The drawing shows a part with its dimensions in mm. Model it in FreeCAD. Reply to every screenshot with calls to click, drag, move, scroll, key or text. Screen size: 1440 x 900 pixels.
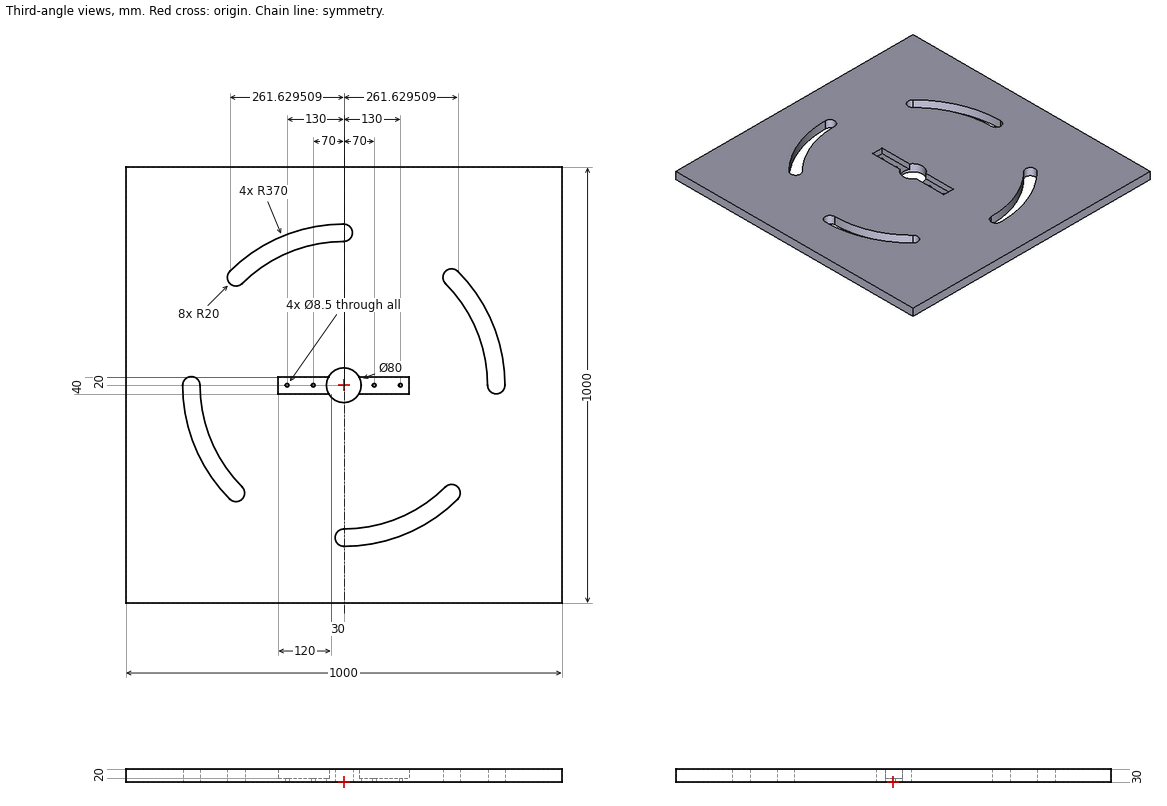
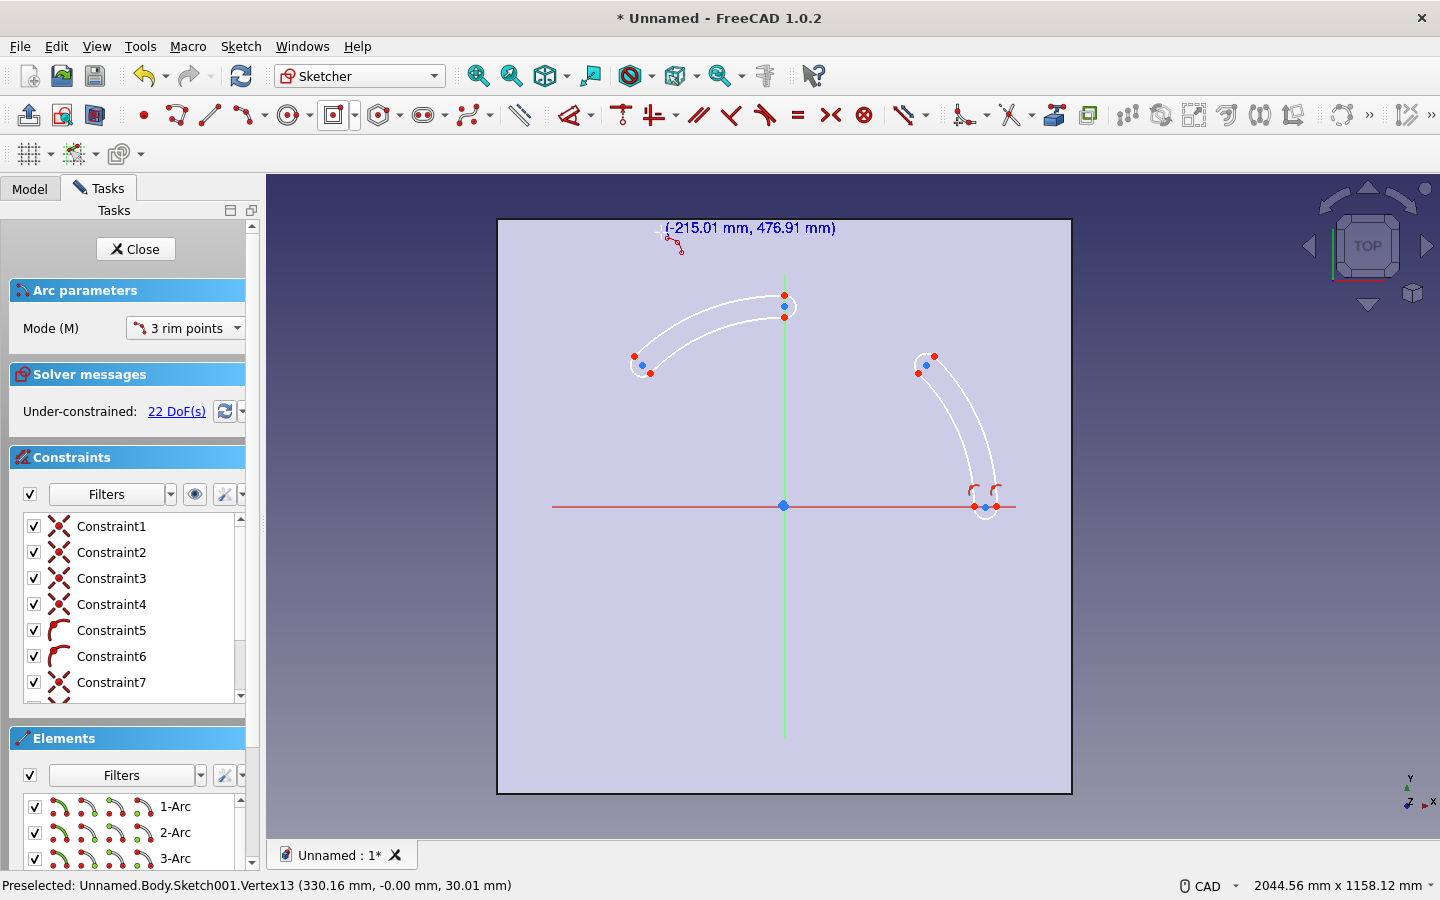
click(785, 696)
click(785, 719)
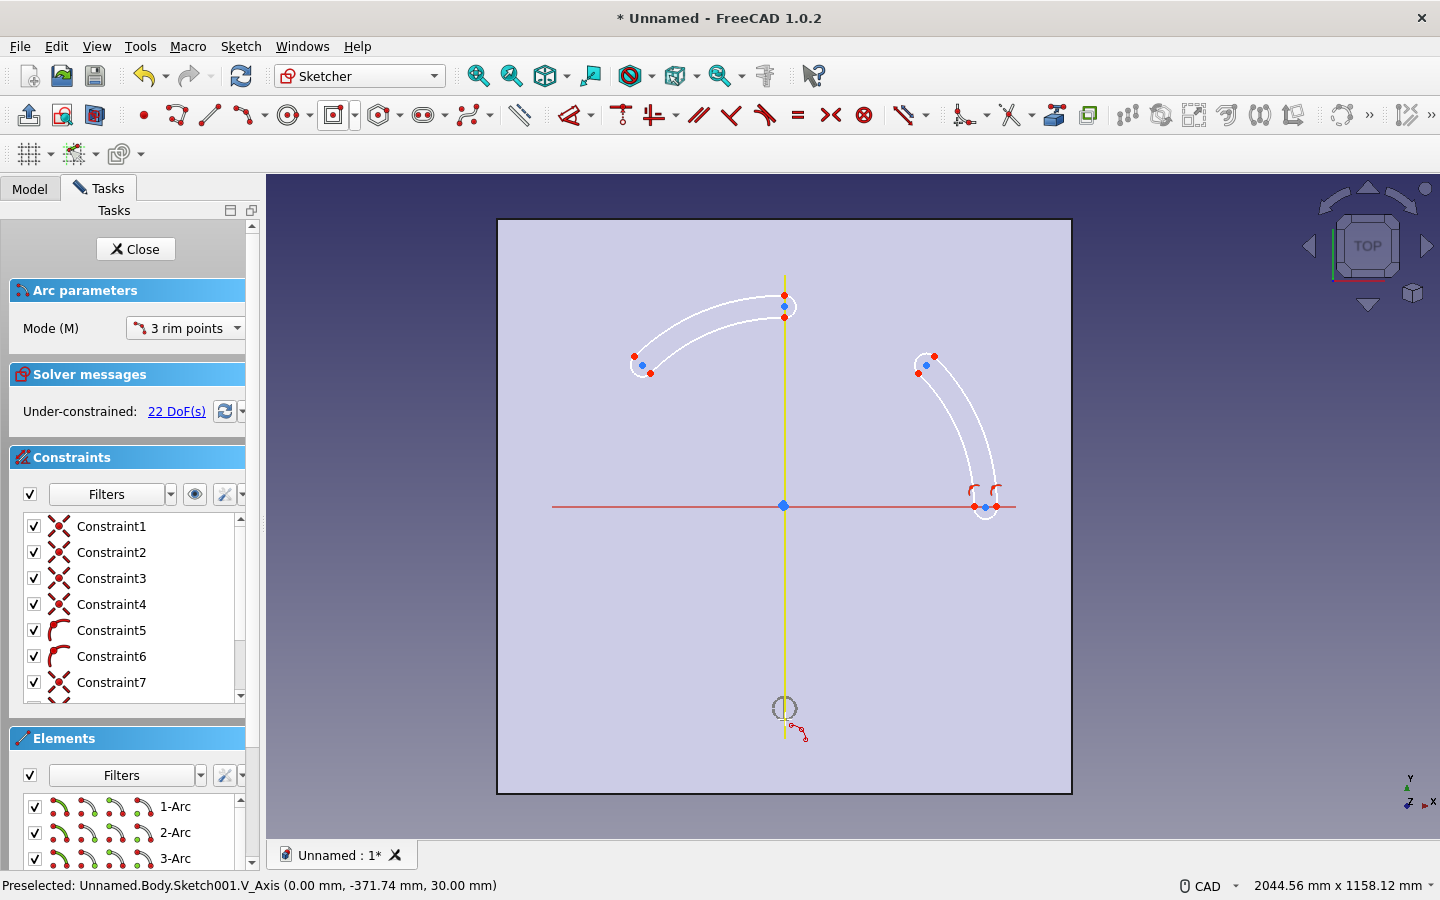
scroll(773, 708, up, 2)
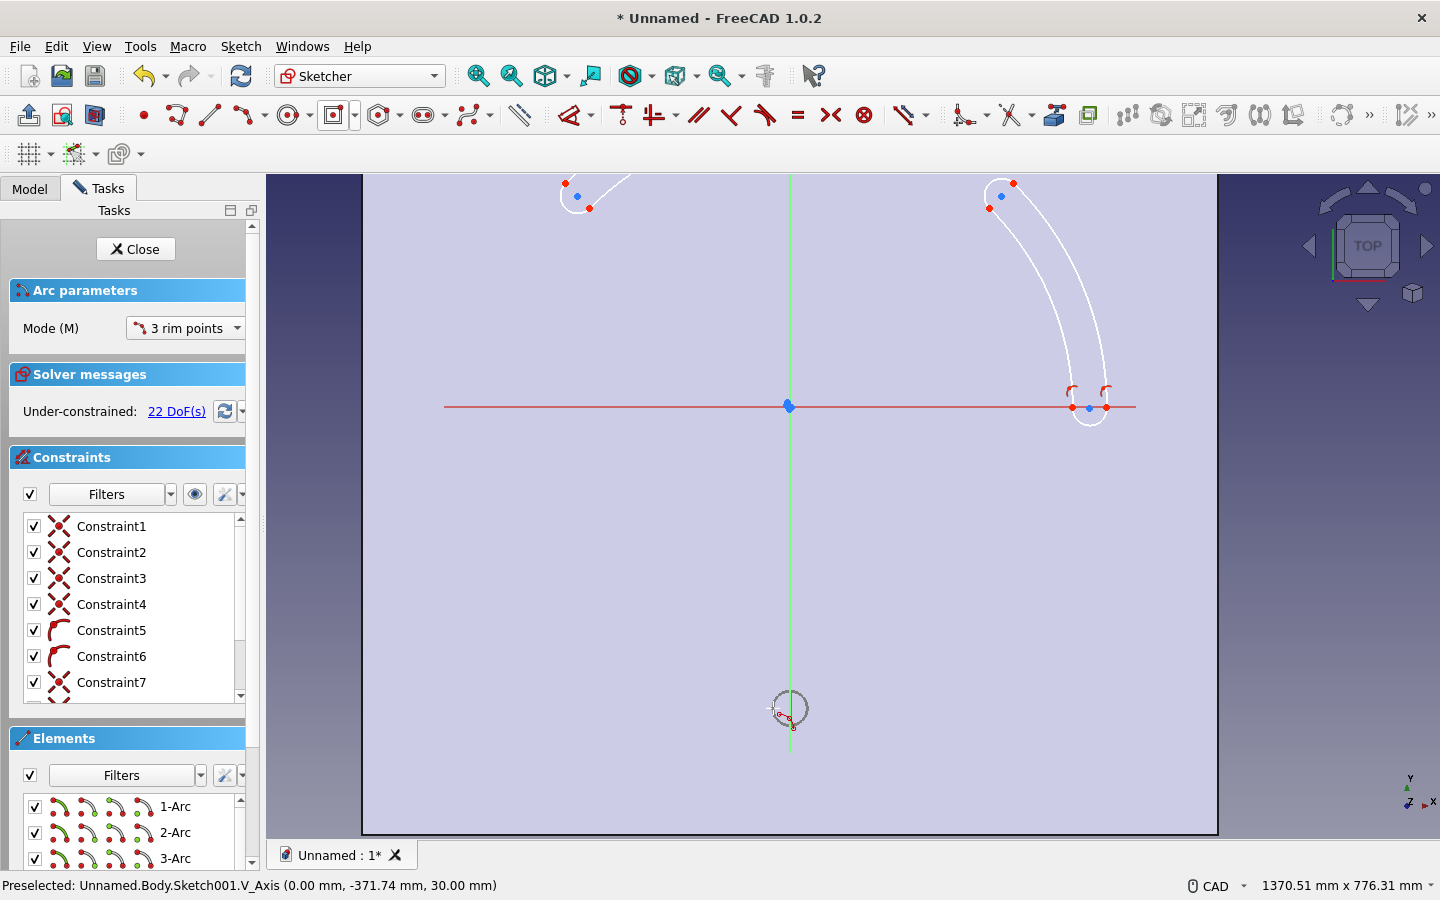
click(773, 707)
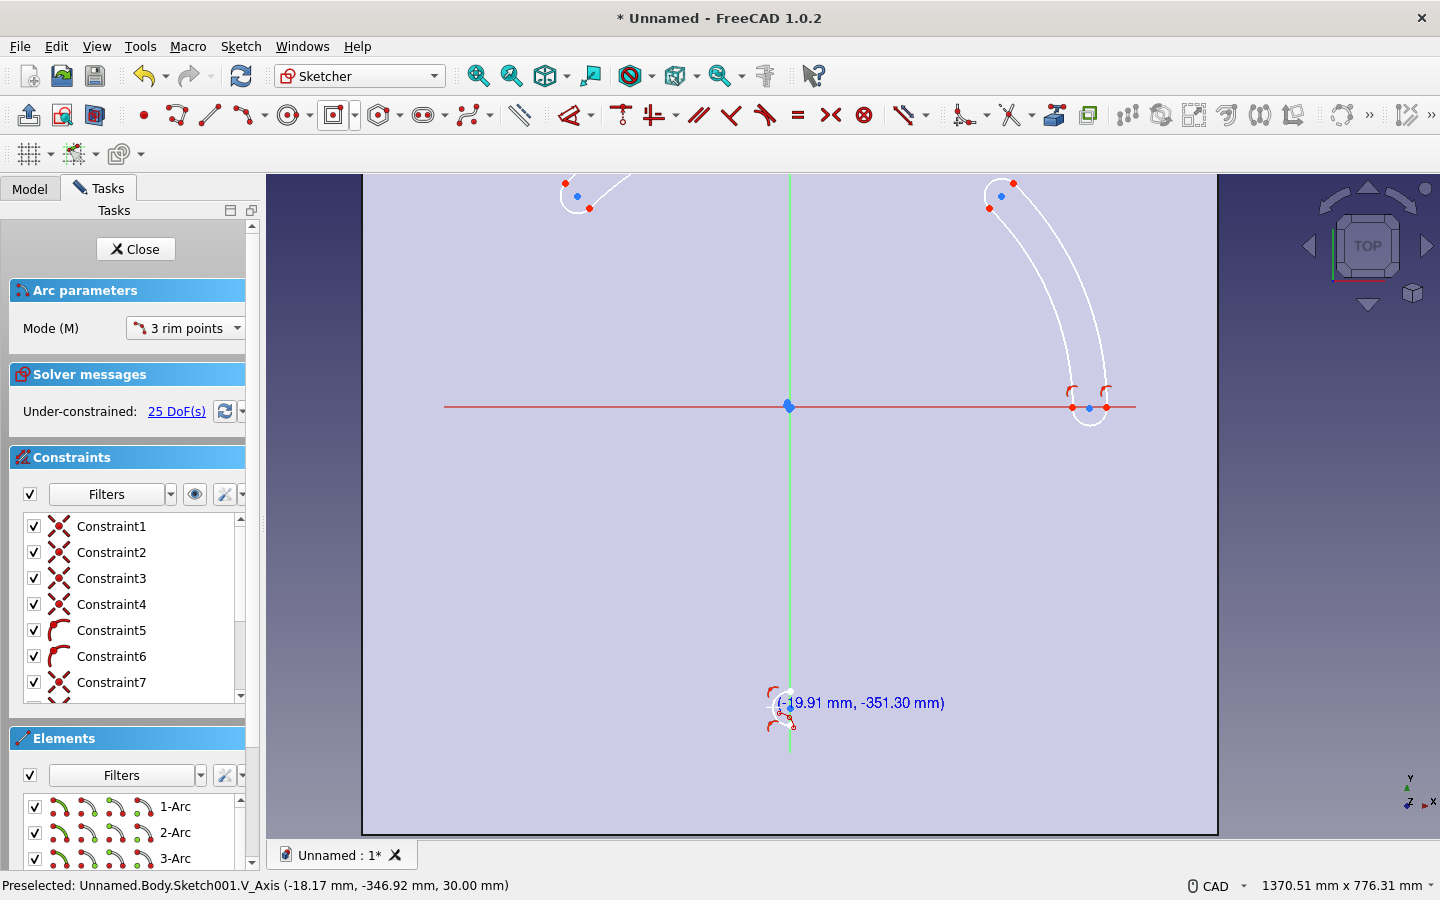
click(790, 726)
click(1014, 631)
click(911, 700)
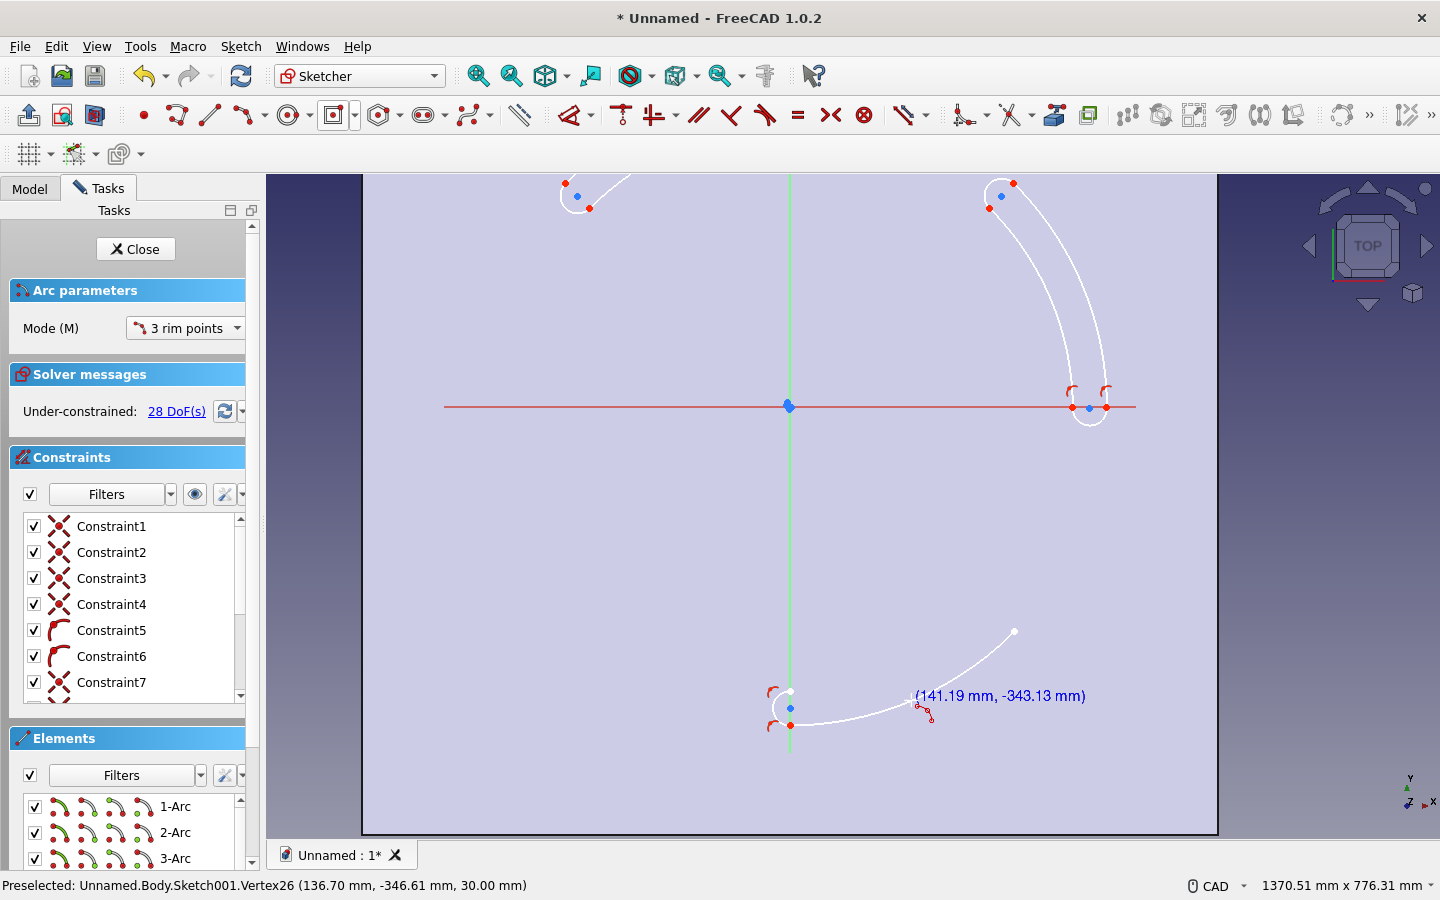
click(1014, 632)
click(990, 607)
click(1014, 607)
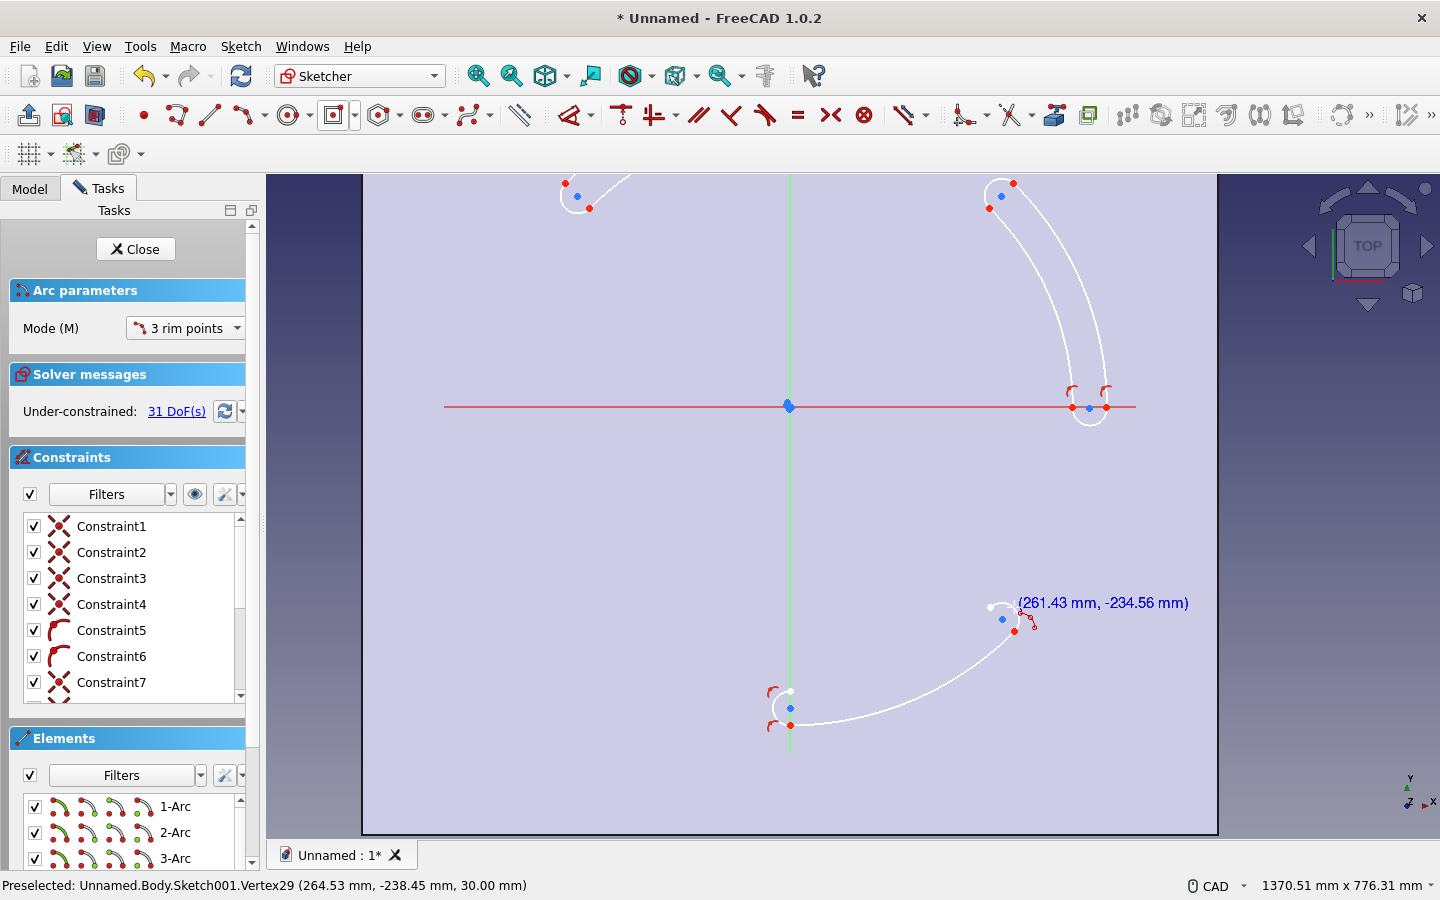
click(990, 608)
click(790, 691)
click(898, 668)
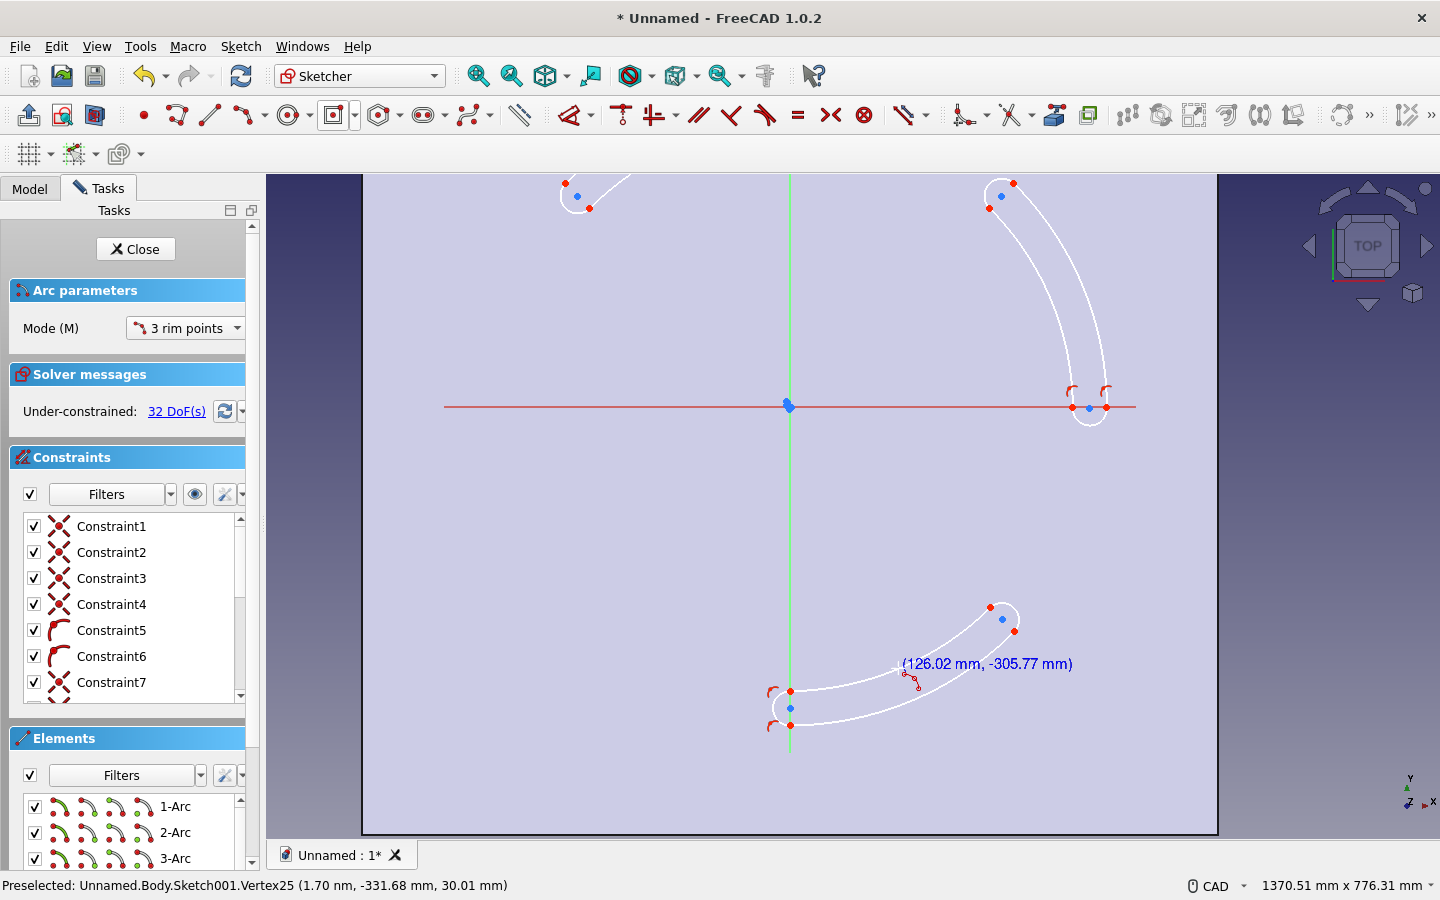
click(507, 407)
click(473, 407)
click(490, 390)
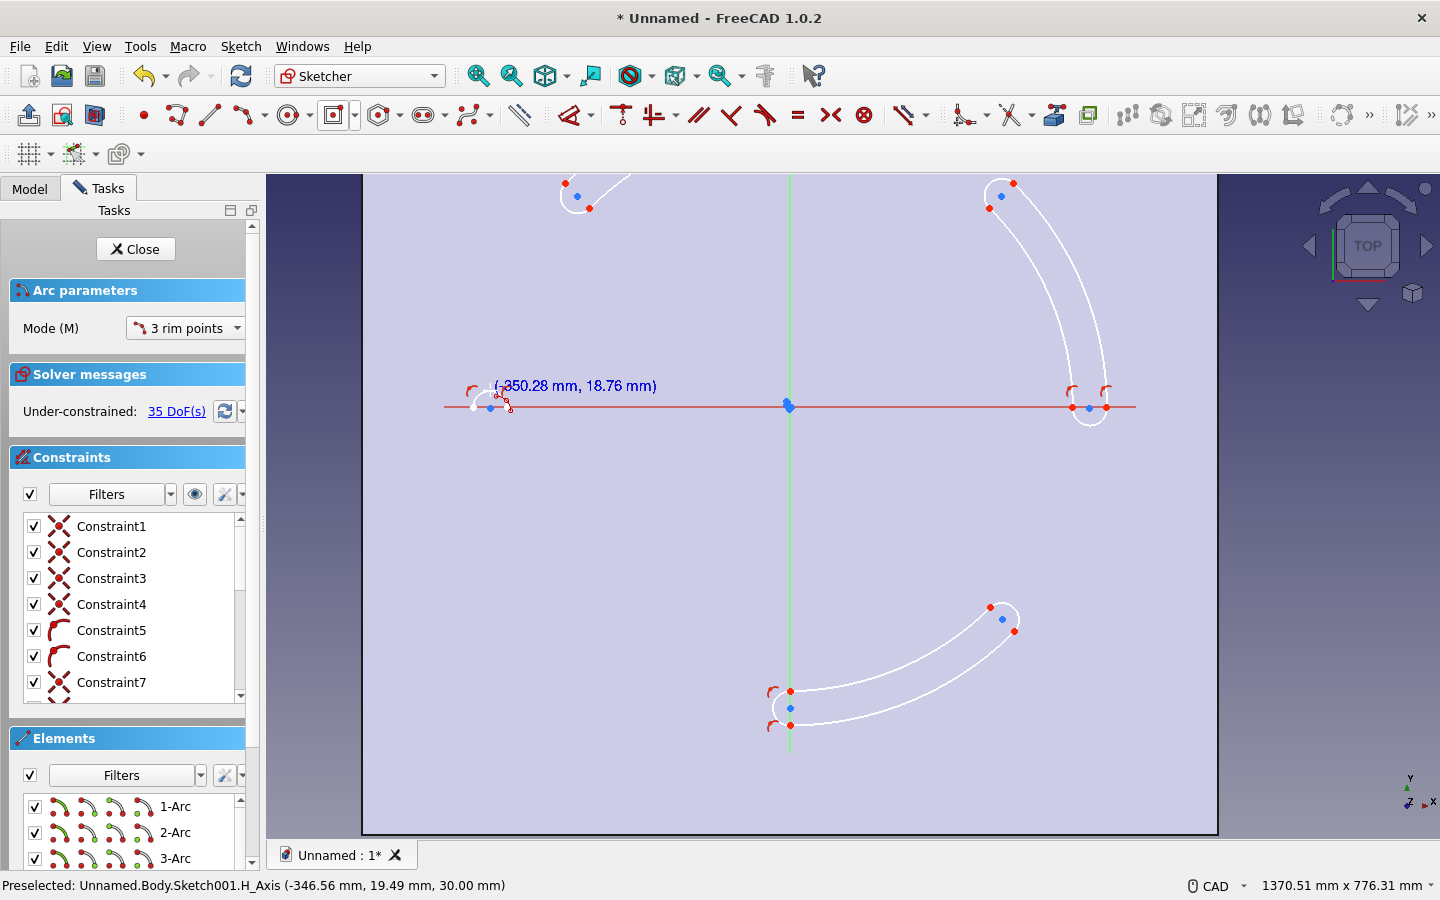
click(473, 407)
click(566, 631)
click(497, 528)